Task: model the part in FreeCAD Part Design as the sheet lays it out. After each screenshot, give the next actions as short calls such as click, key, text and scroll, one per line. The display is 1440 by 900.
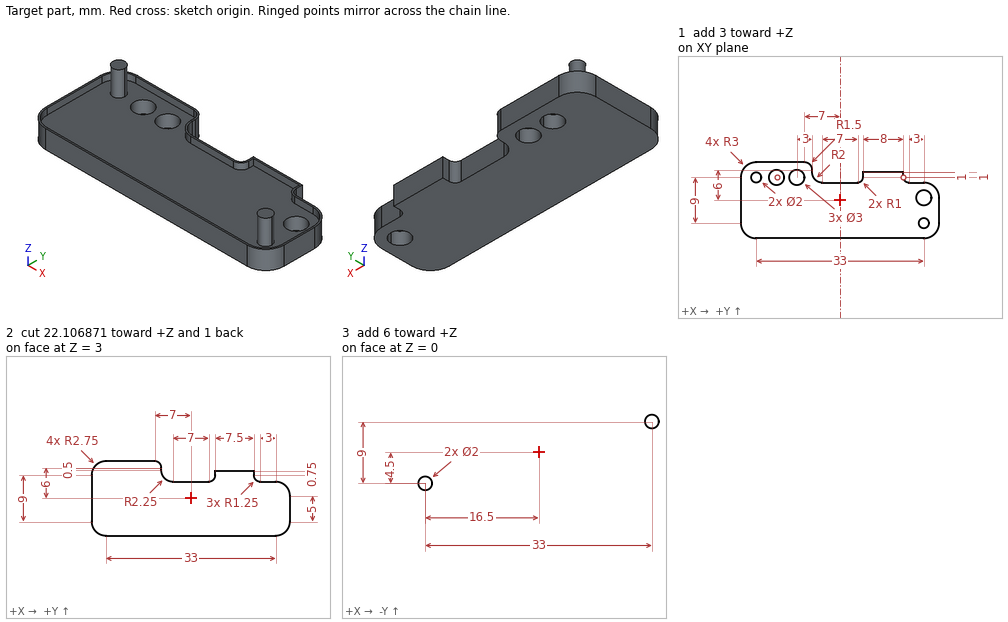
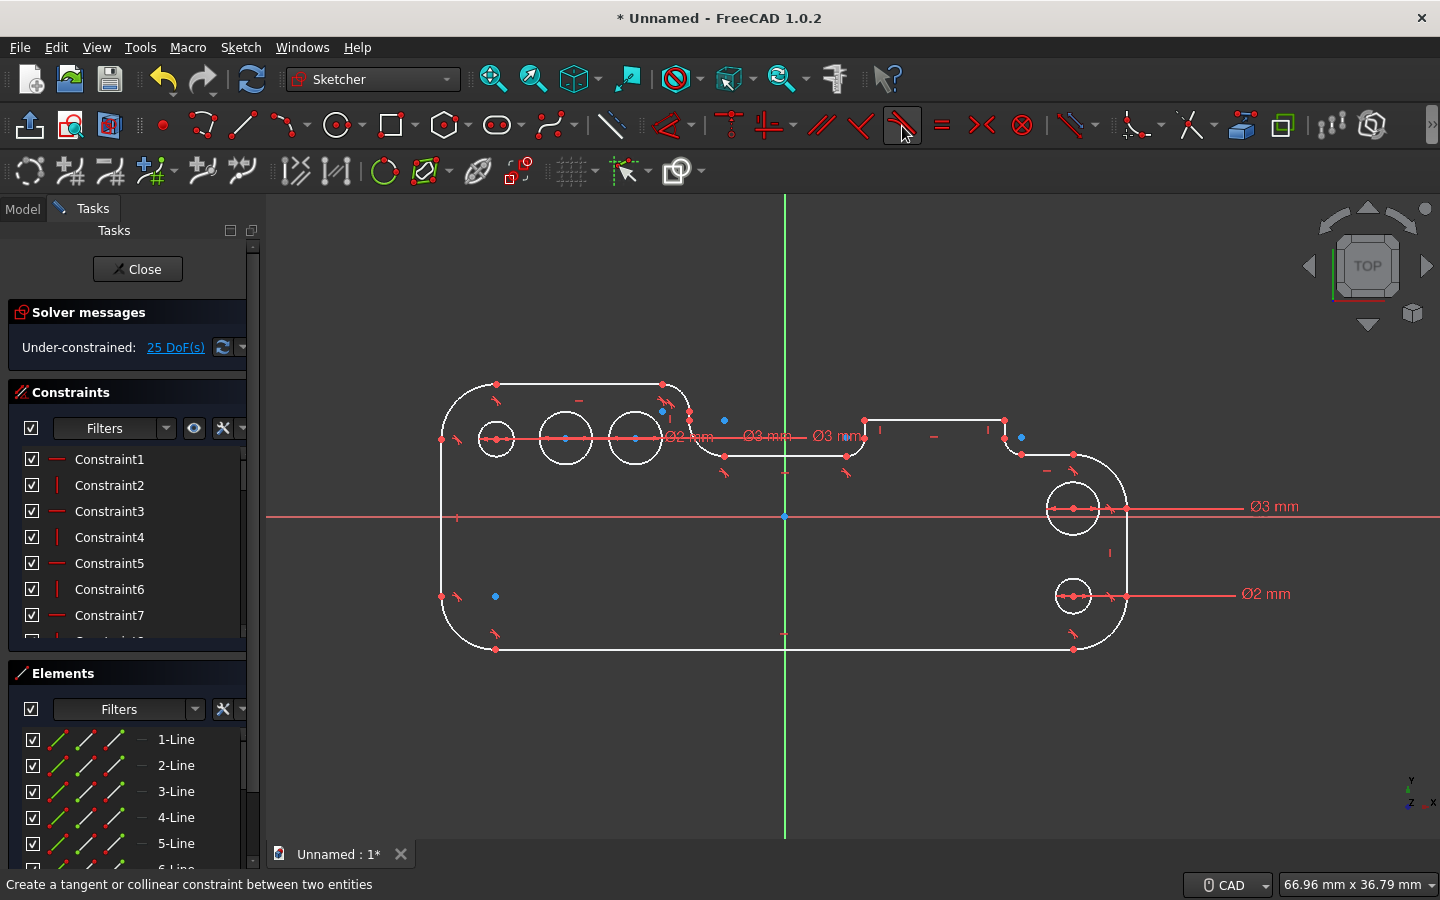
click(1058, 455)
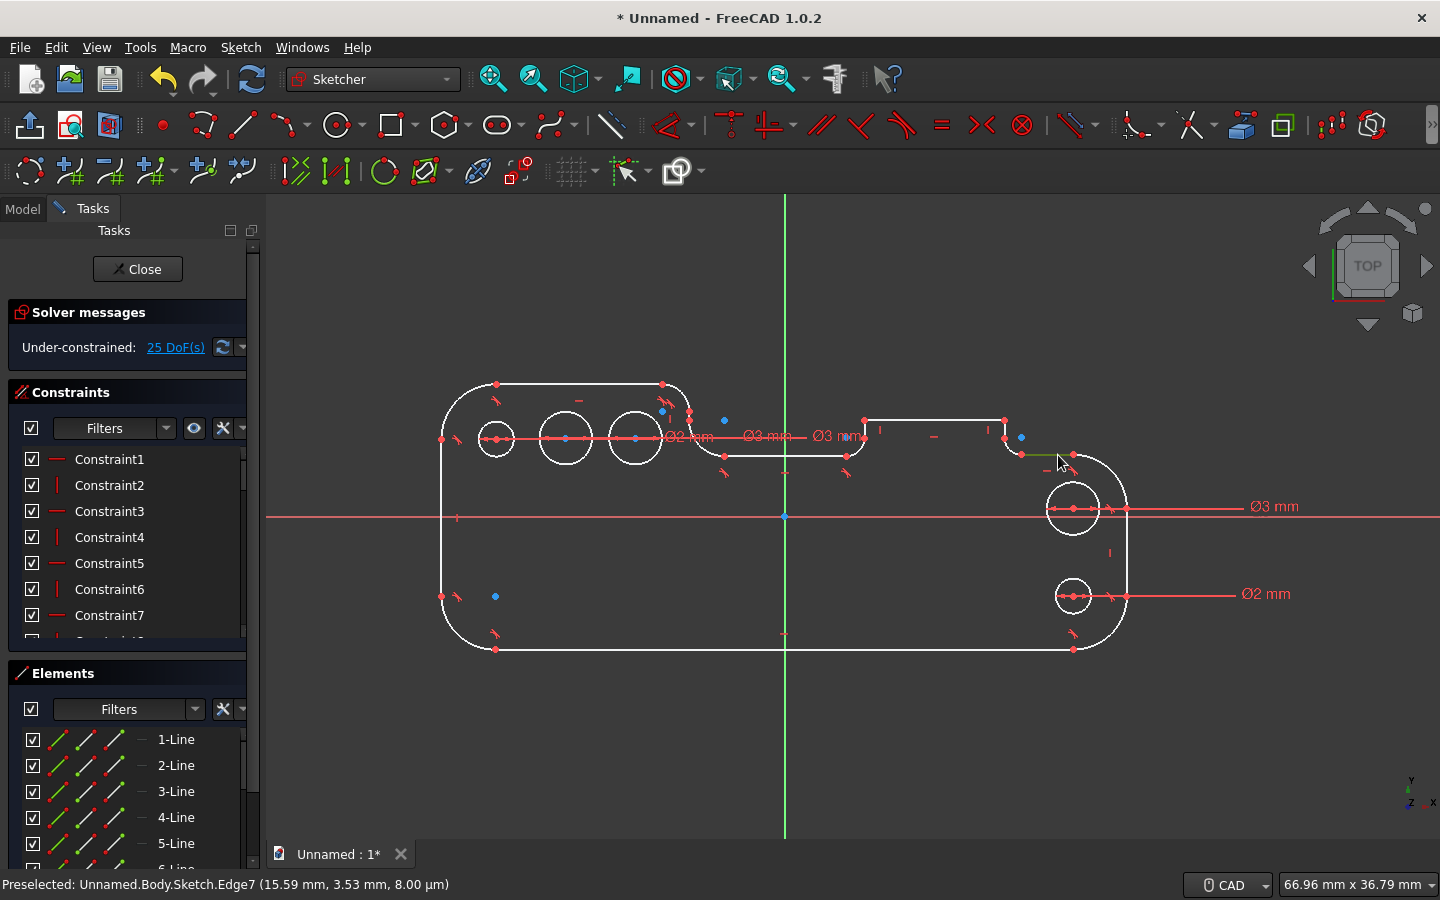
click(1010, 450)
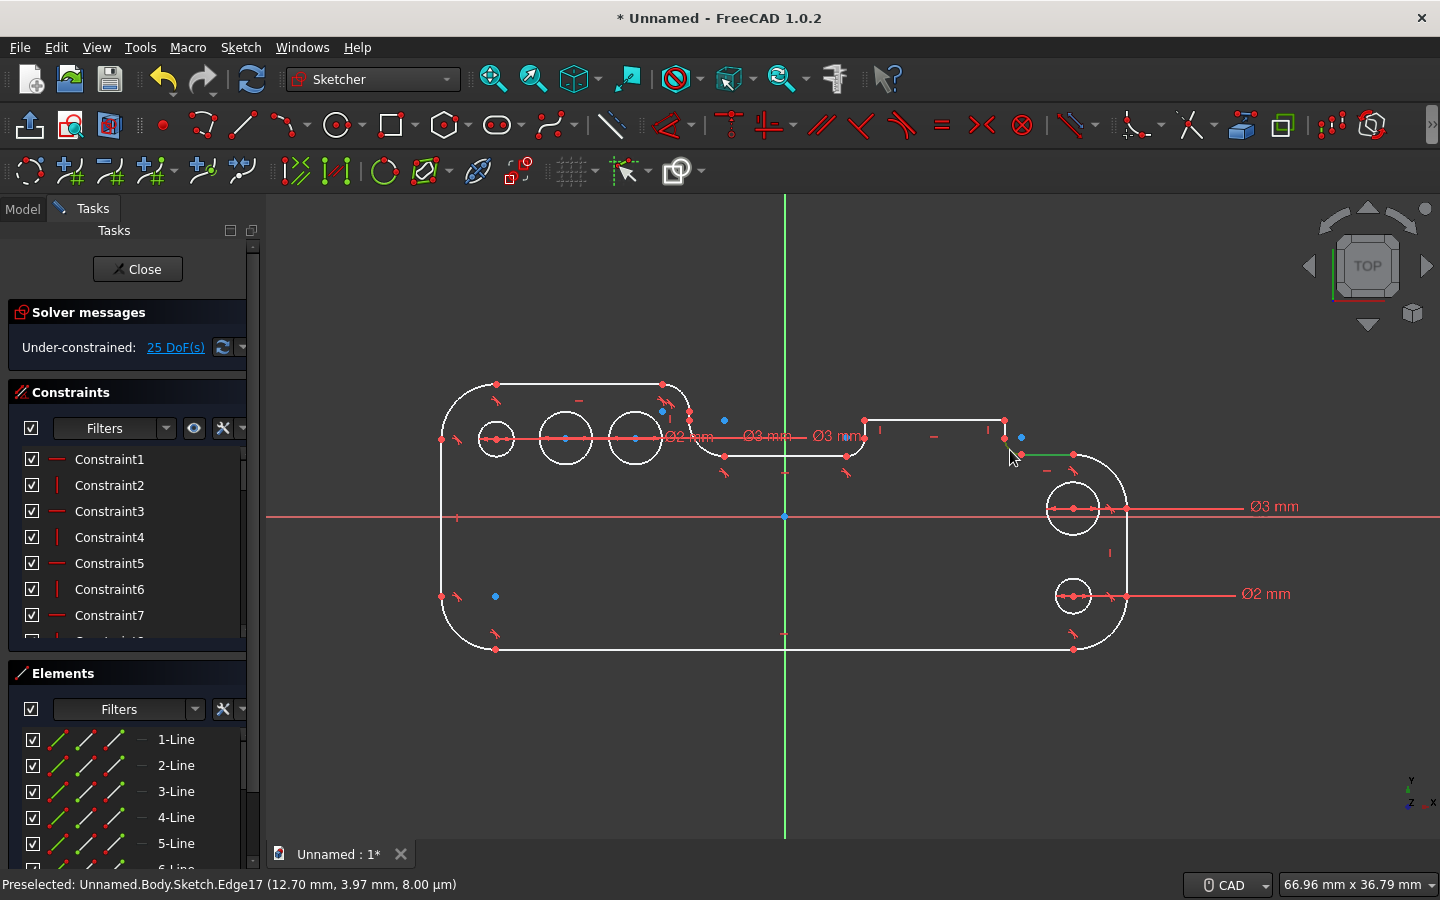
click(902, 126)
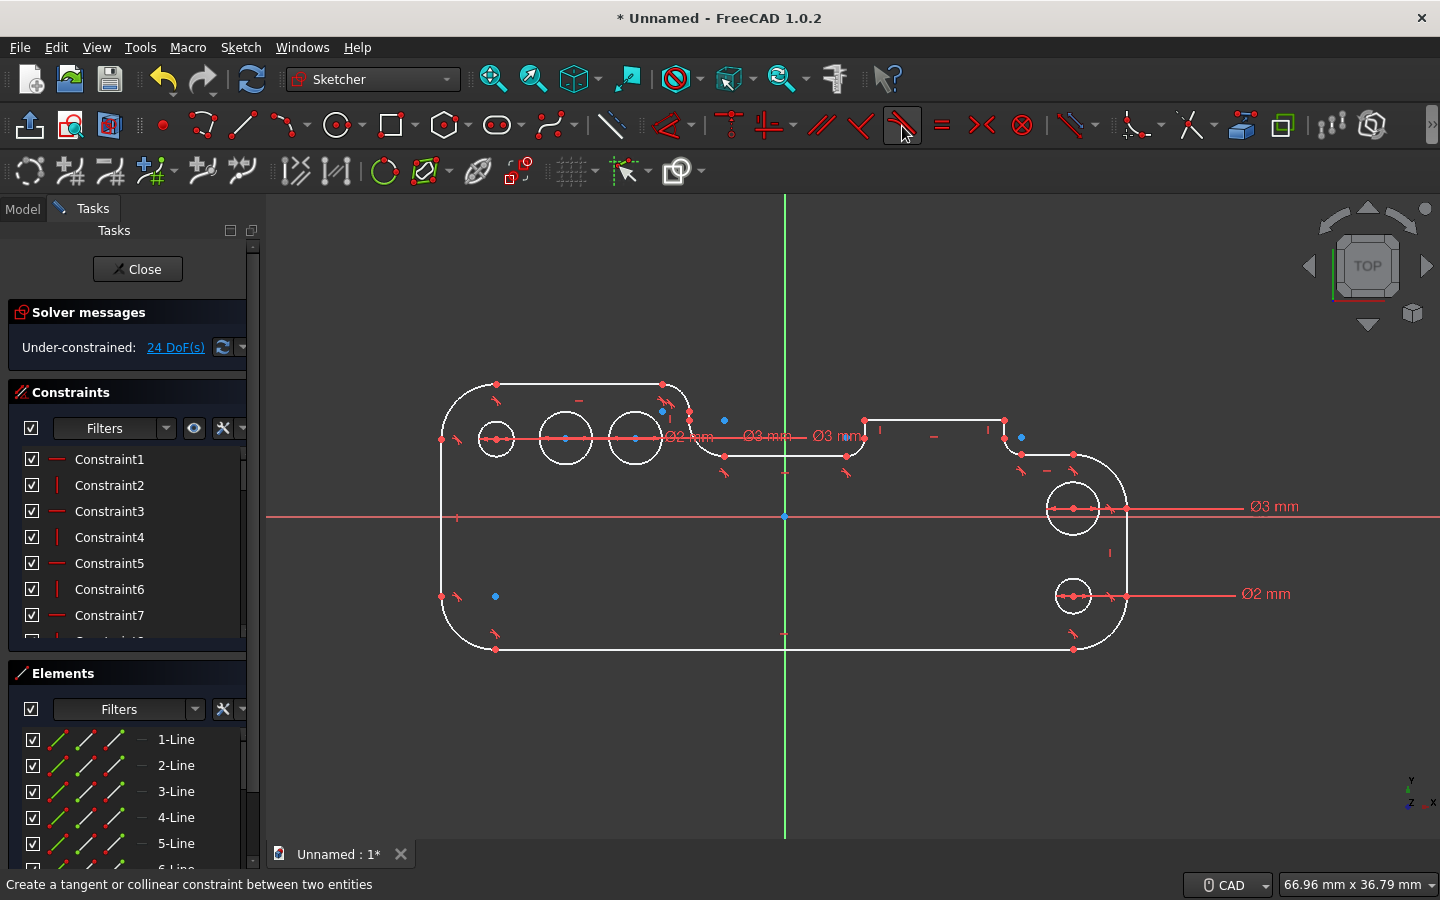
scroll(1004, 429, up, 3)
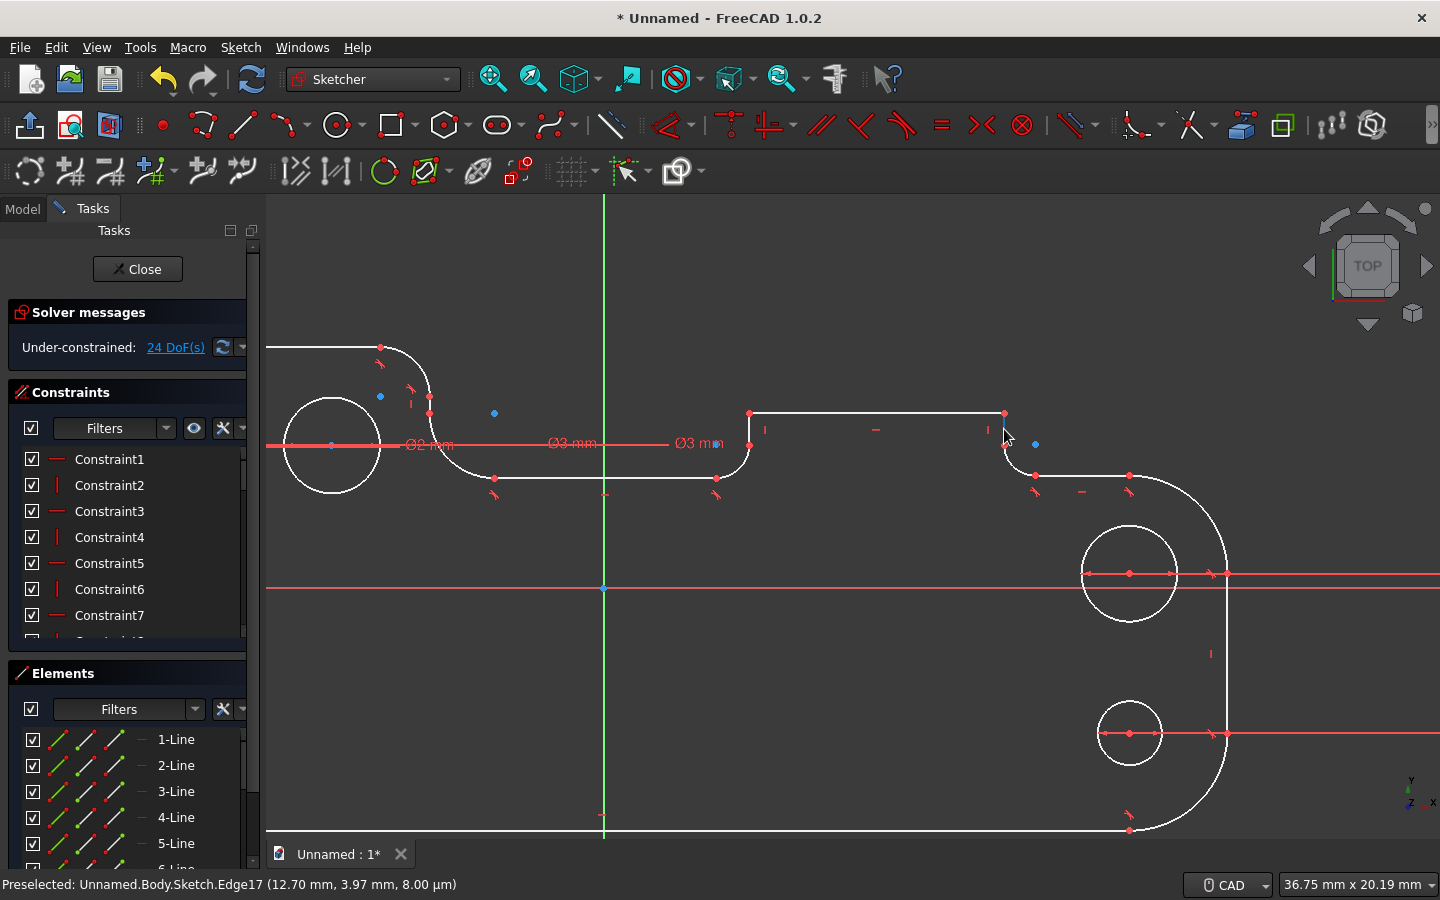
click(1004, 429)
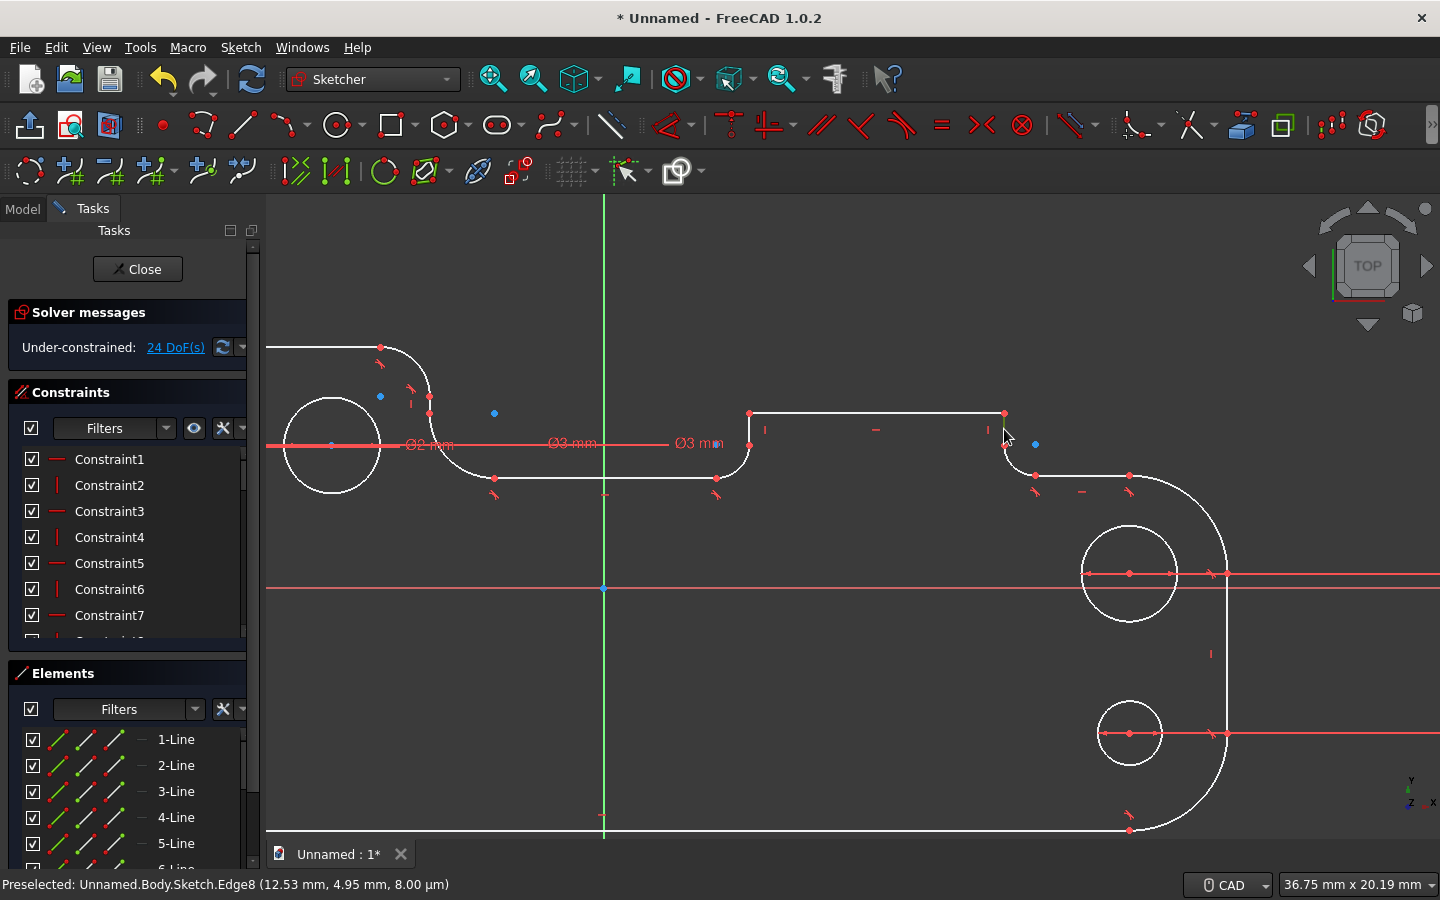
click(1008, 459)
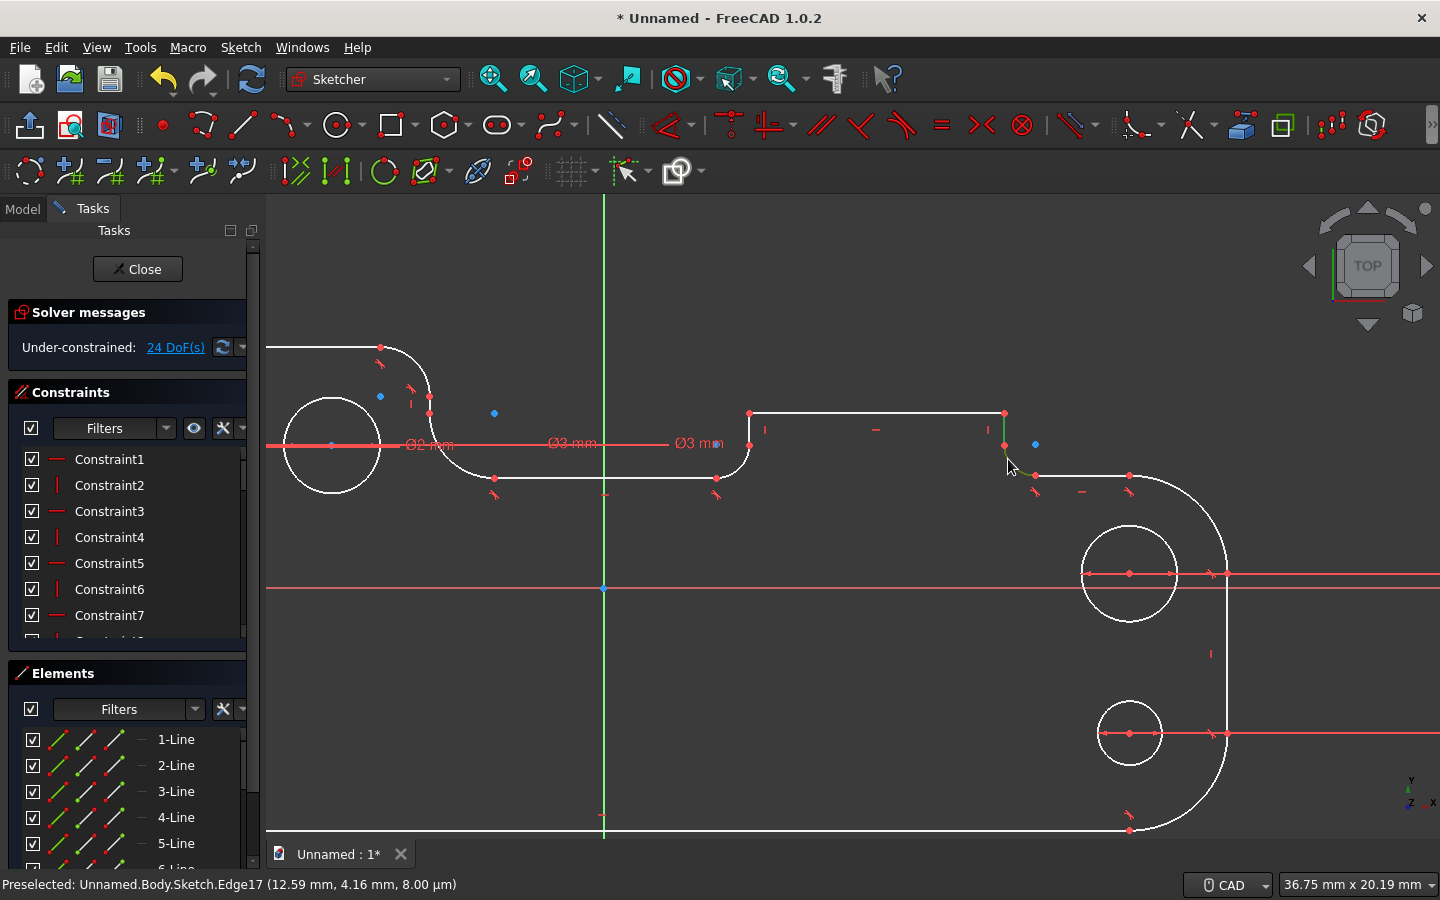
key(t)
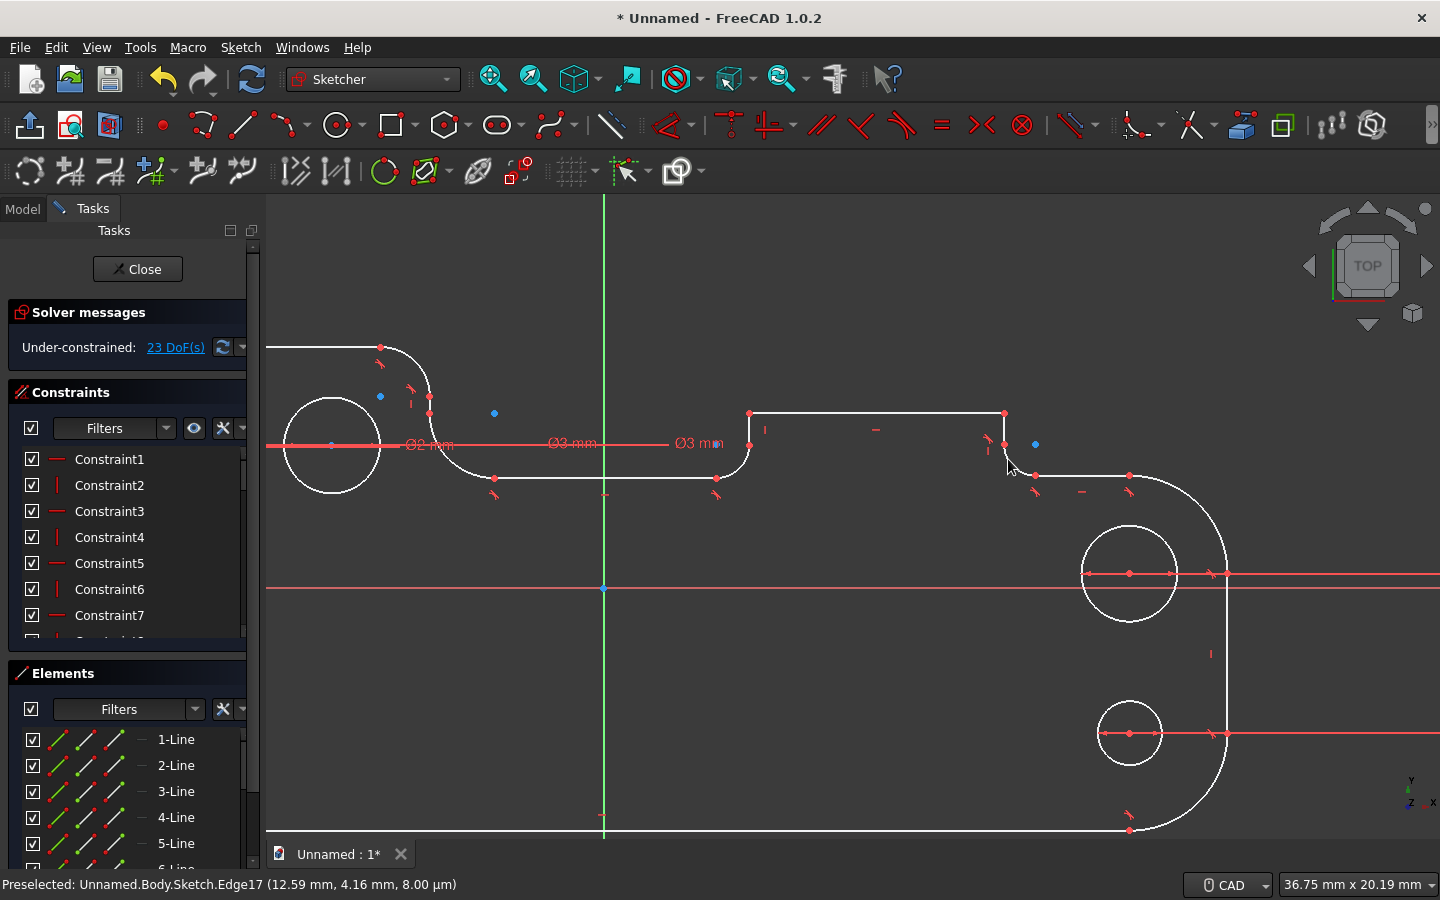
scroll(749, 423, up, 2)